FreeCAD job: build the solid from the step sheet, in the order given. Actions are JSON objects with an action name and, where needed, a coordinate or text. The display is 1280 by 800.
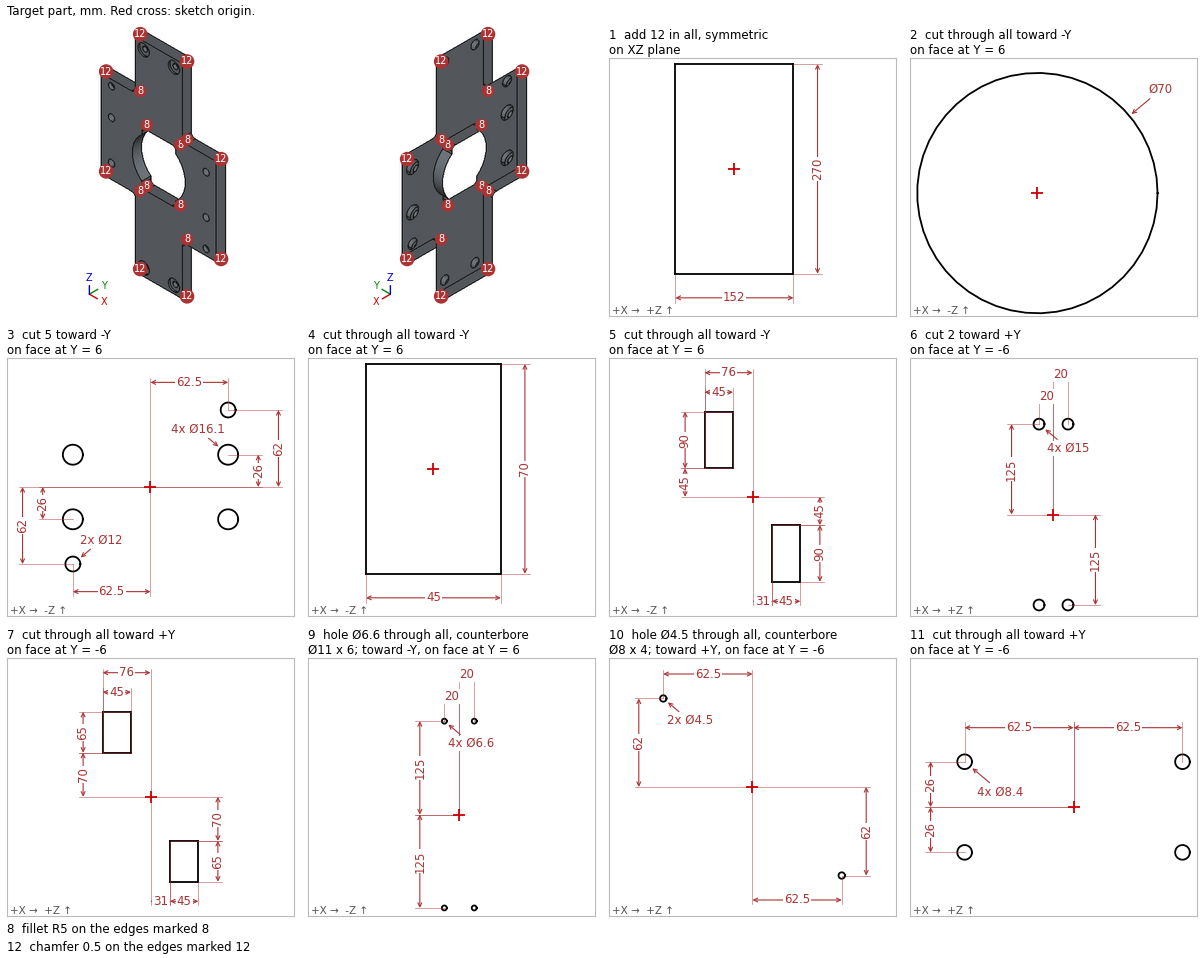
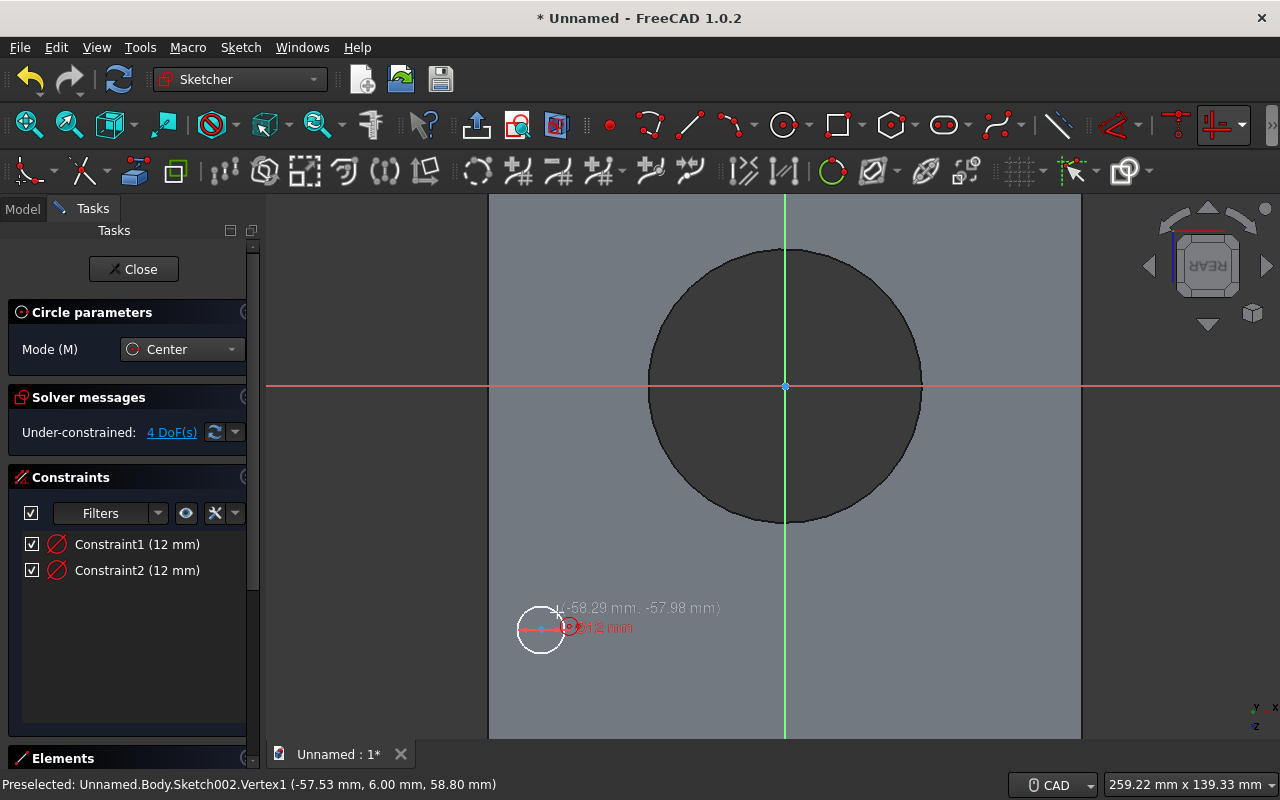
{"action": "left_click", "coordinate": [1029, 284]}
{"action": "mouse_move", "coordinate": [1052, 262]}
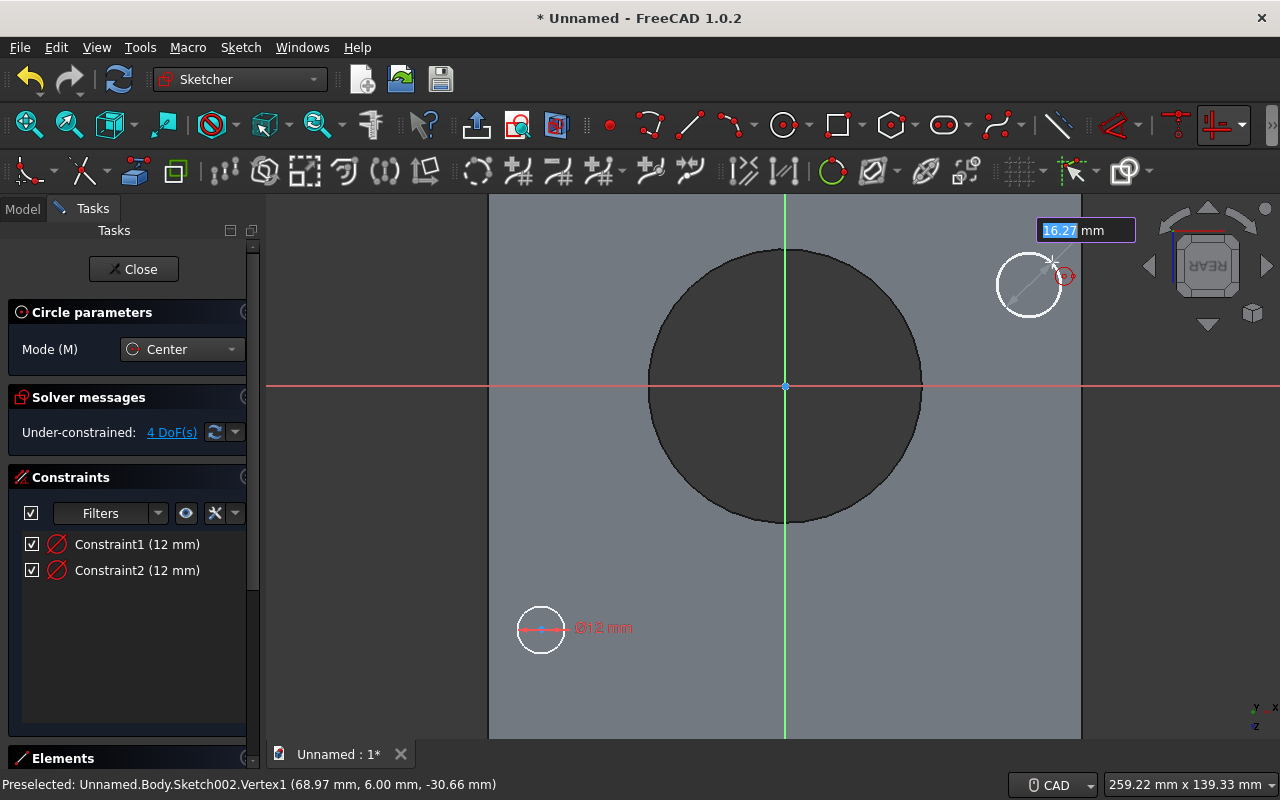
{"action": "type", "text": "16.1"}
{"action": "key", "text": "Return"}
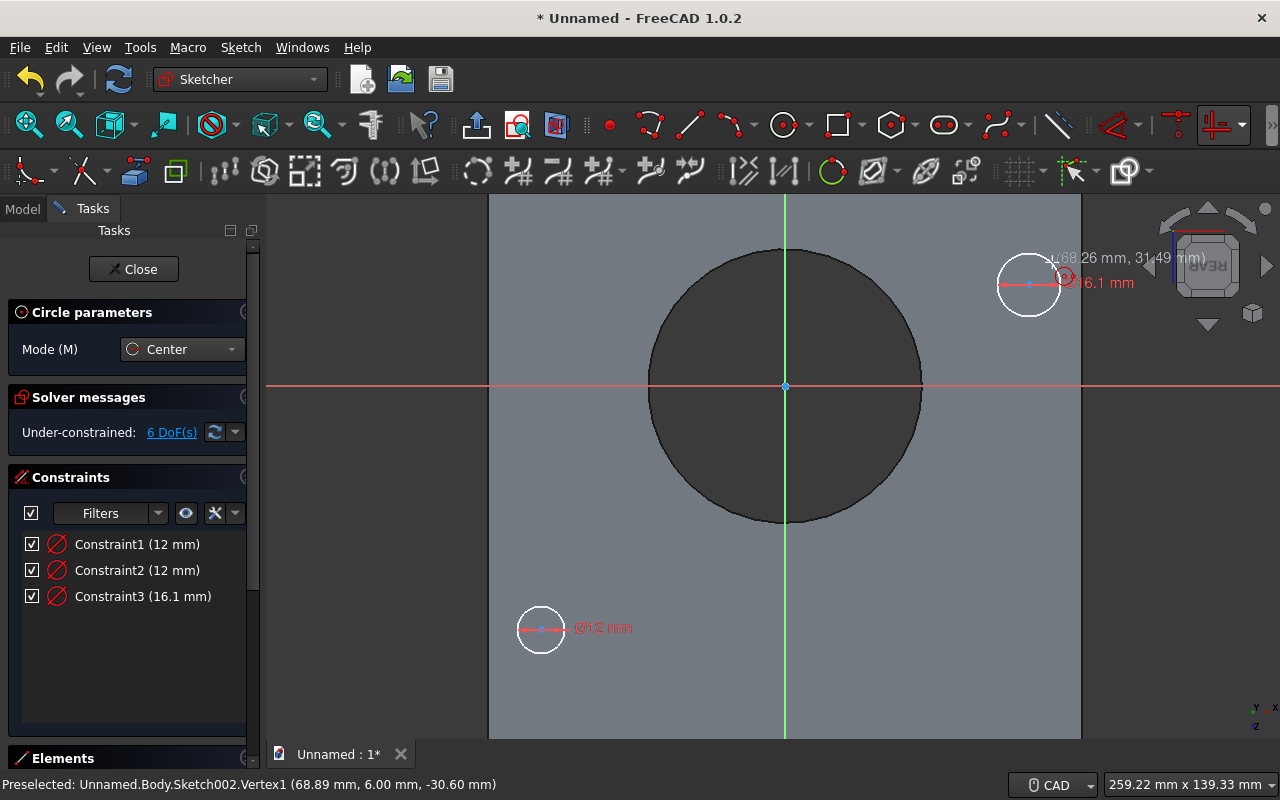
{"action": "left_click", "coordinate": [541, 284]}
{"action": "mouse_move", "coordinate": [563, 262]}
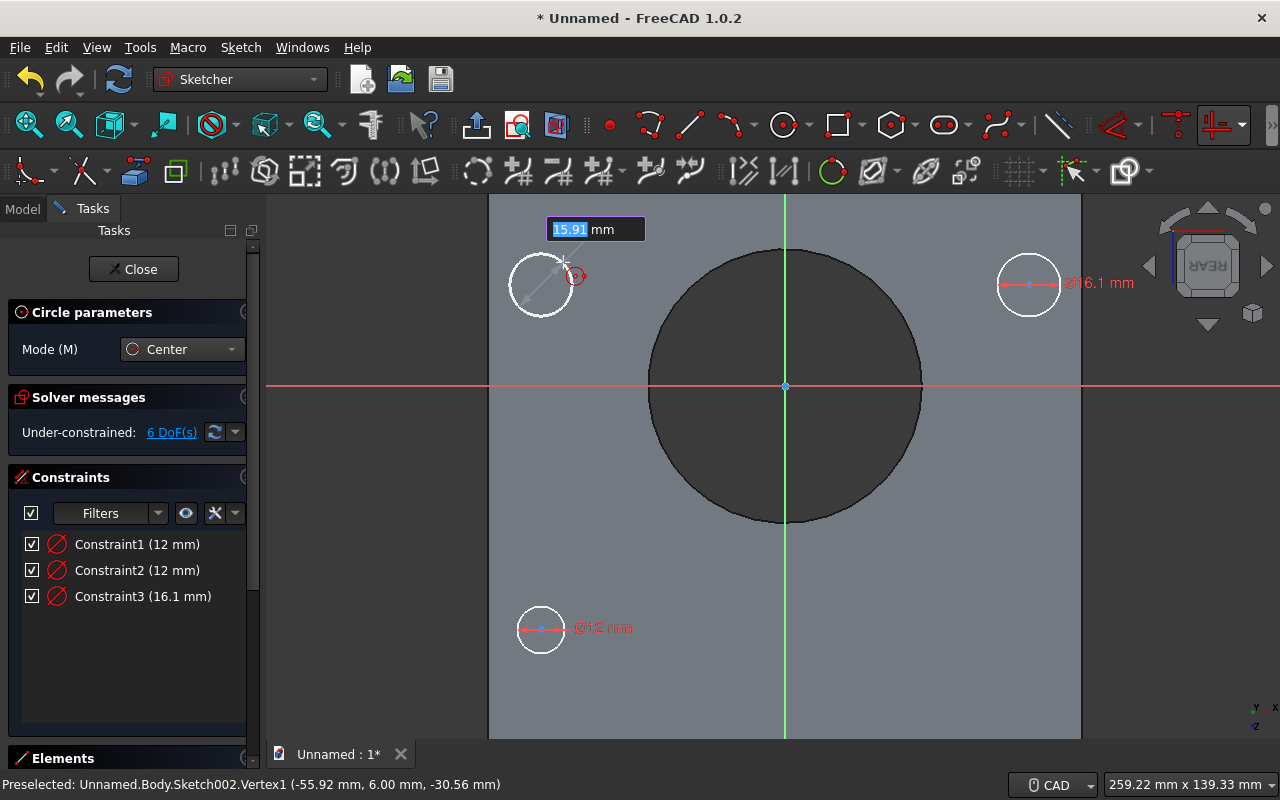
{"action": "type", "text": "16.1"}
{"action": "key", "text": "Return"}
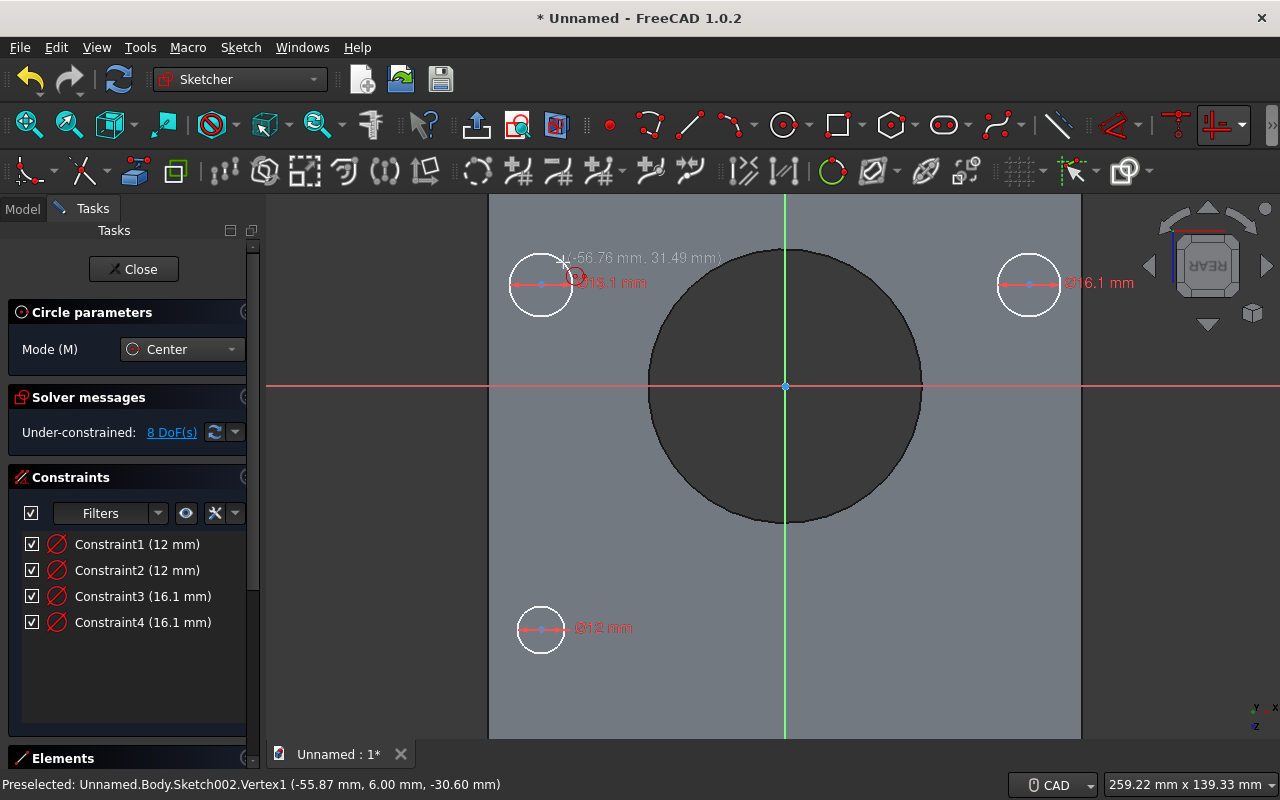
{"action": "left_click", "coordinate": [541, 488]}
{"action": "mouse_move", "coordinate": [563, 466]}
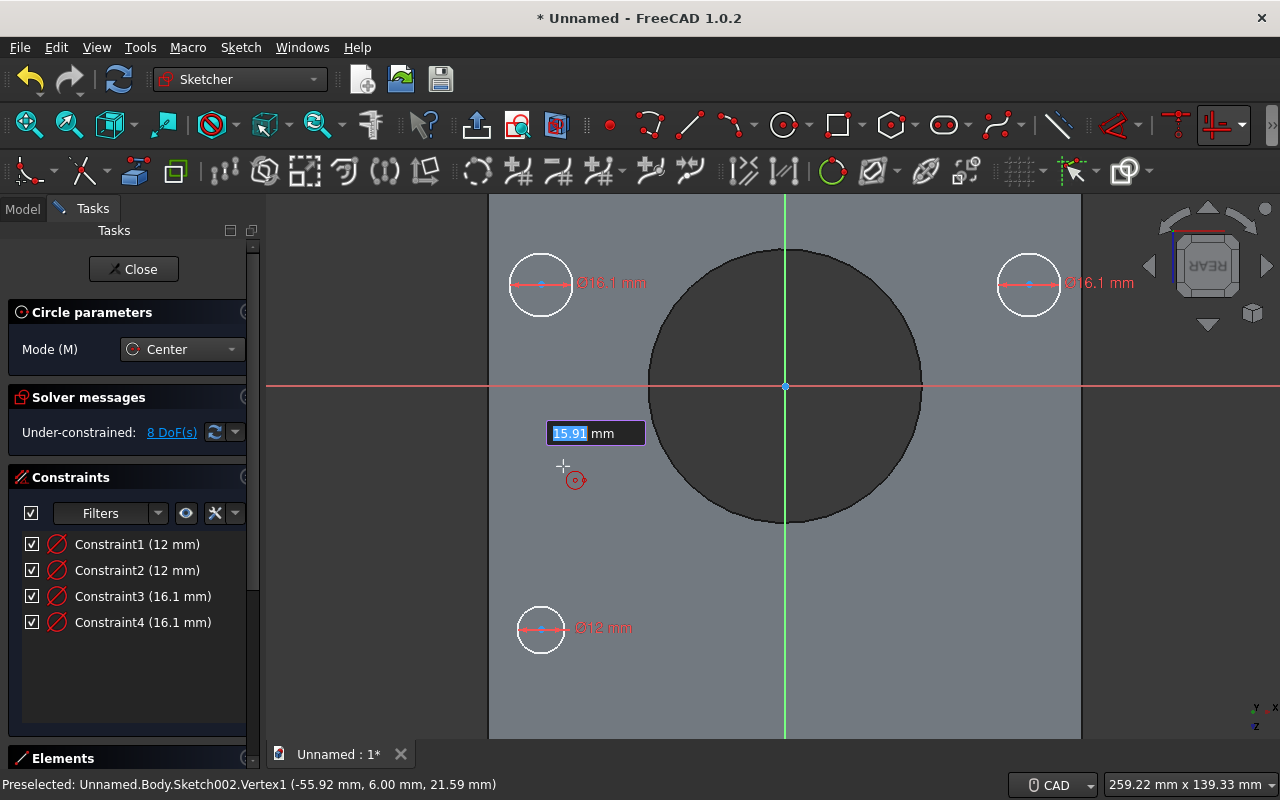
{"action": "type", "text": "16.1"}
{"action": "key", "text": "Return"}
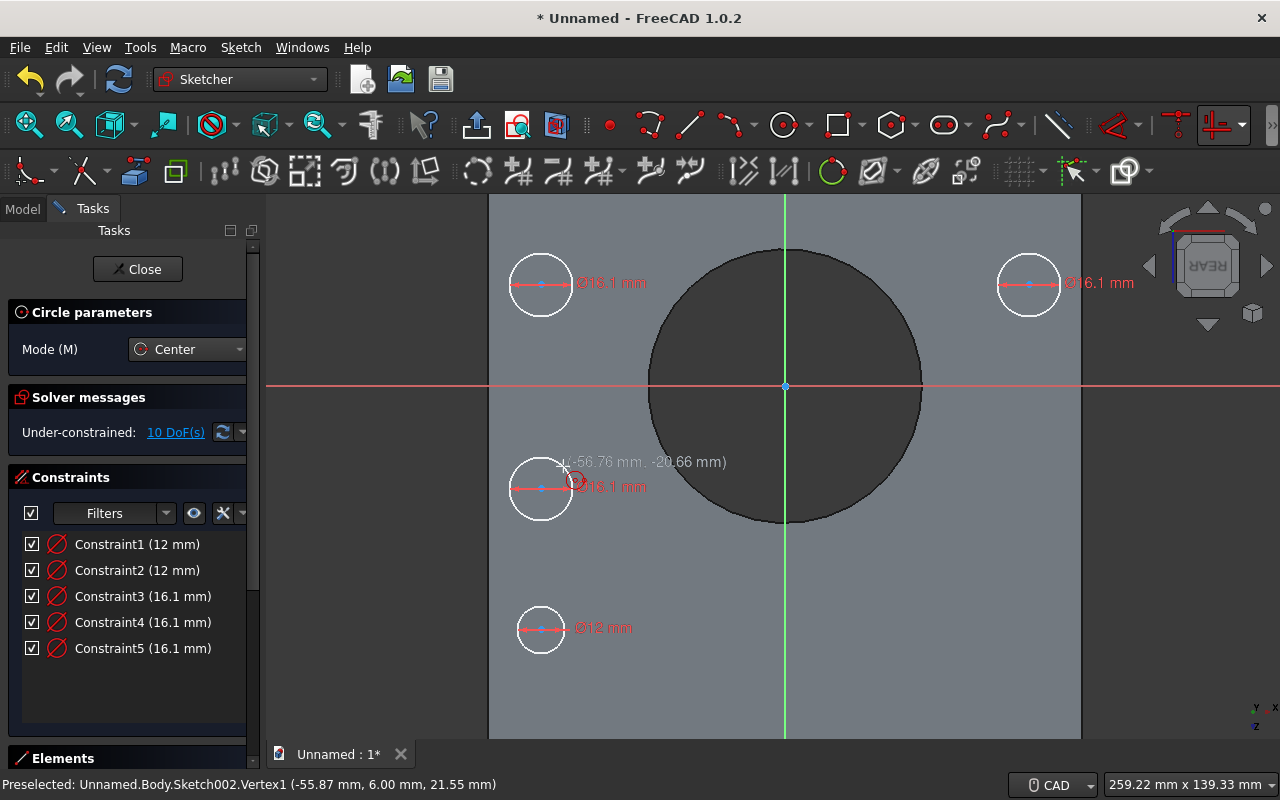
{"action": "left_click", "coordinate": [1029, 488]}
{"action": "mouse_move", "coordinate": [1052, 466]}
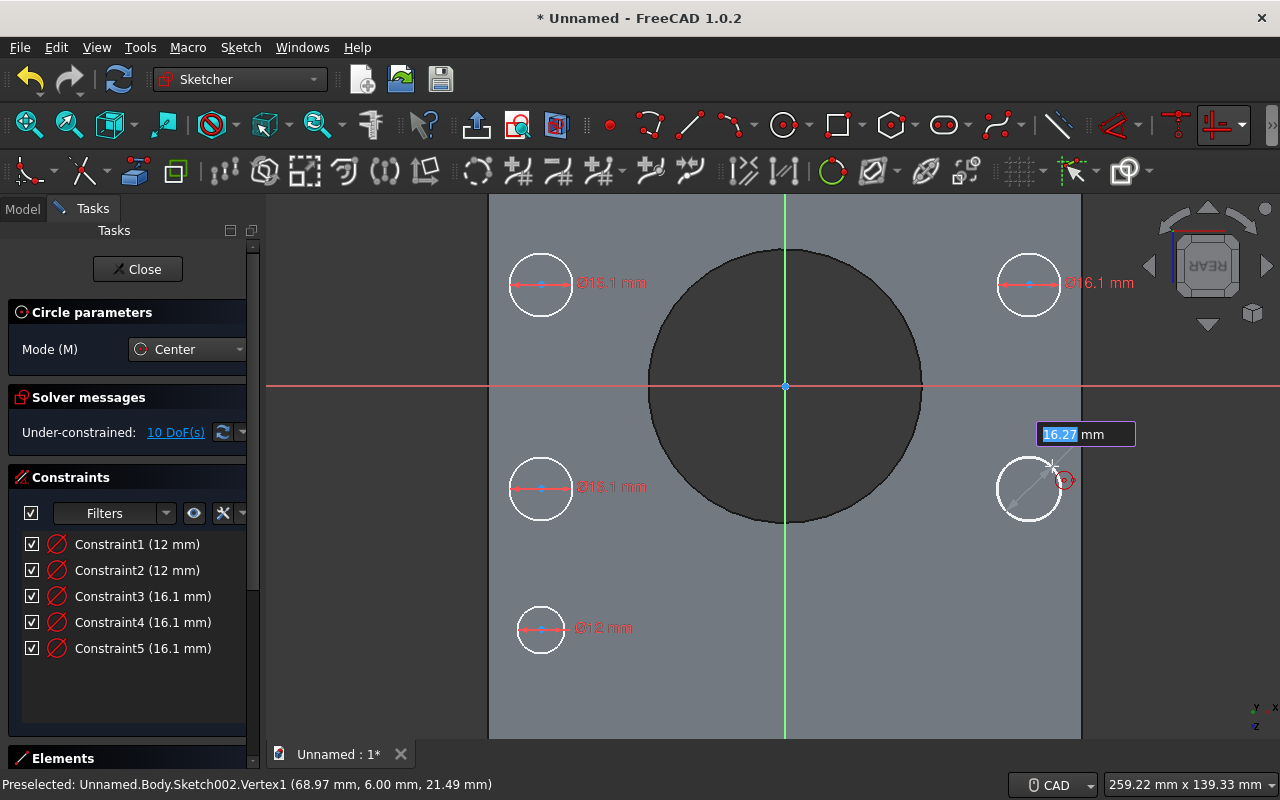
{"action": "type", "text": "16.1"}
{"action": "key", "text": "Return"}
{"action": "key", "text": "Escape"}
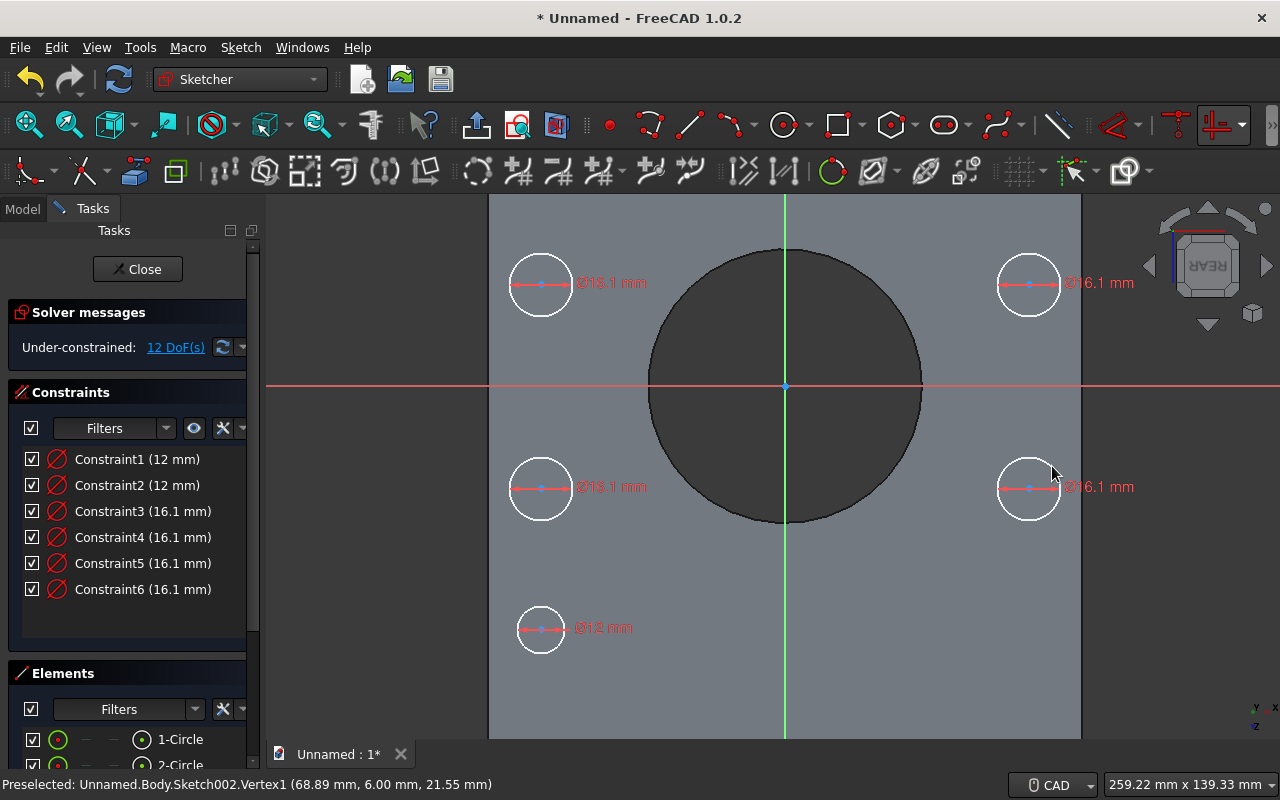
{"action": "scroll", "coordinate": [541, 630], "scroll_direction": "down", "scroll_amount": 2}